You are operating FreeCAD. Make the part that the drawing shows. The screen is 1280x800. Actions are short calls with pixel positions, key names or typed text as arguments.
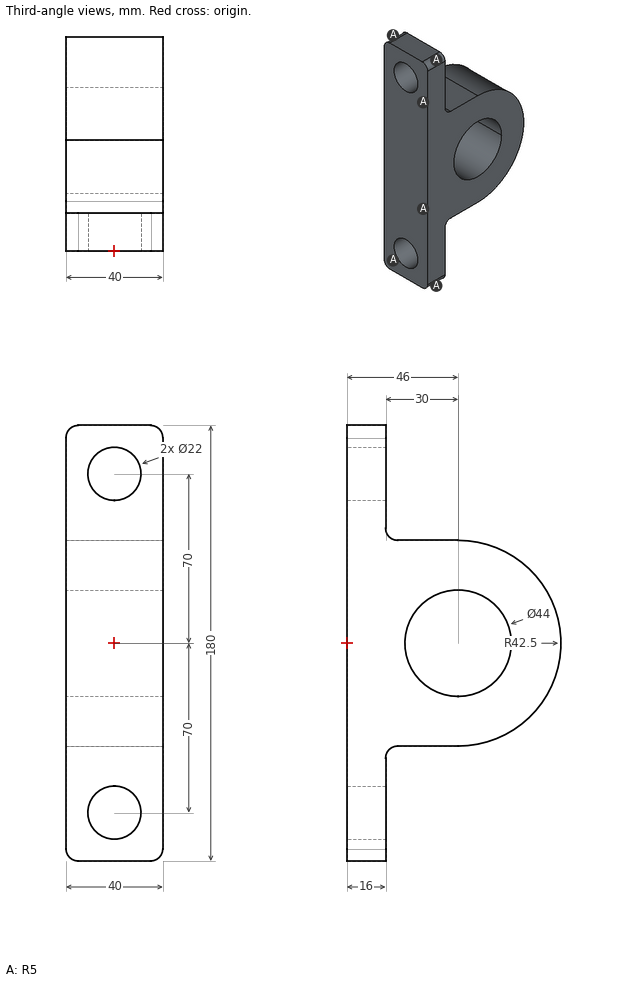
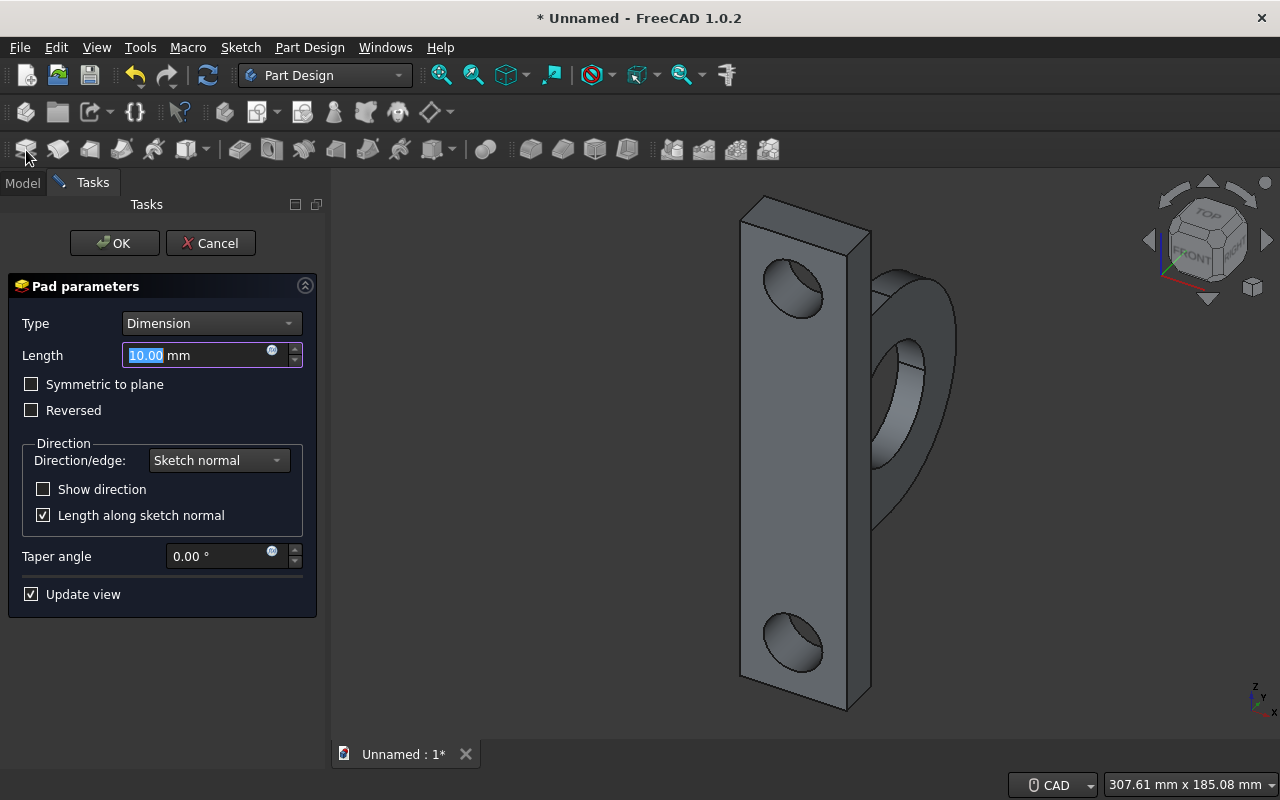
text(40)
key(Tab)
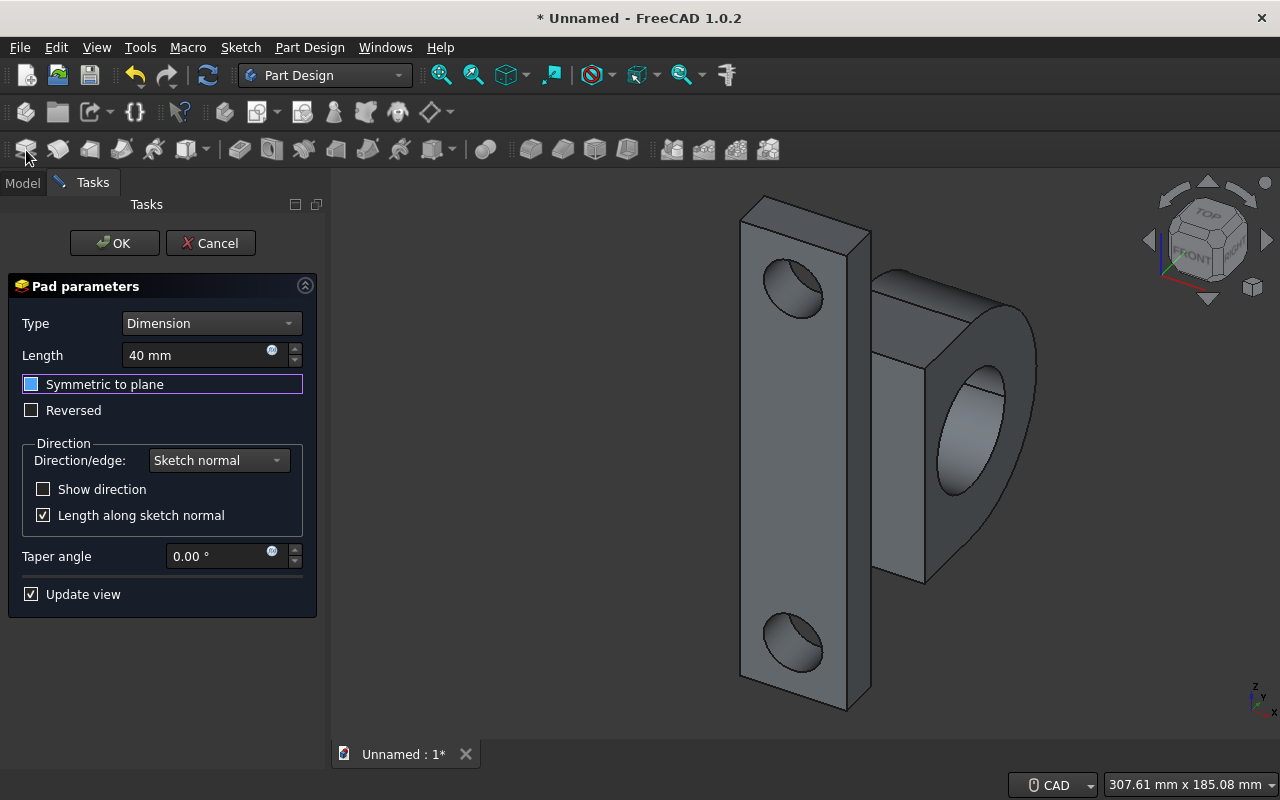
click(30, 384)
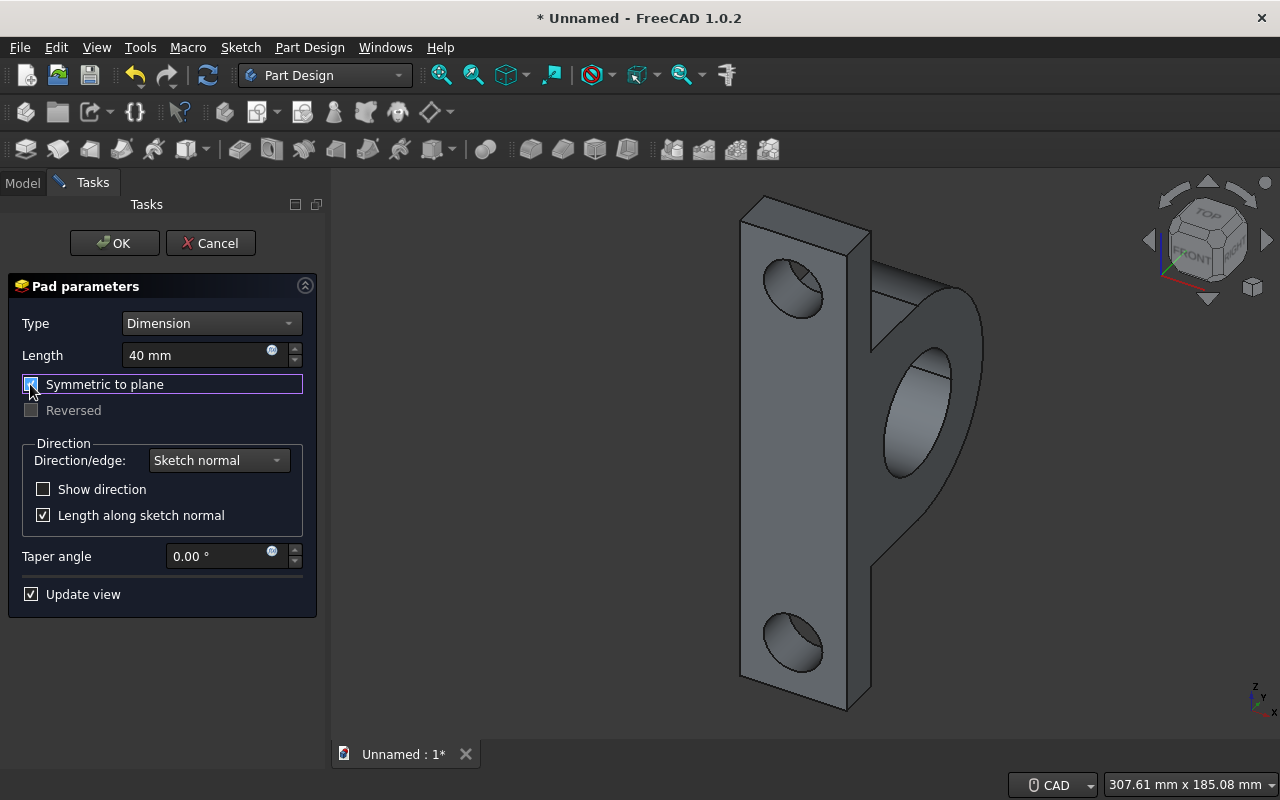
click(115, 243)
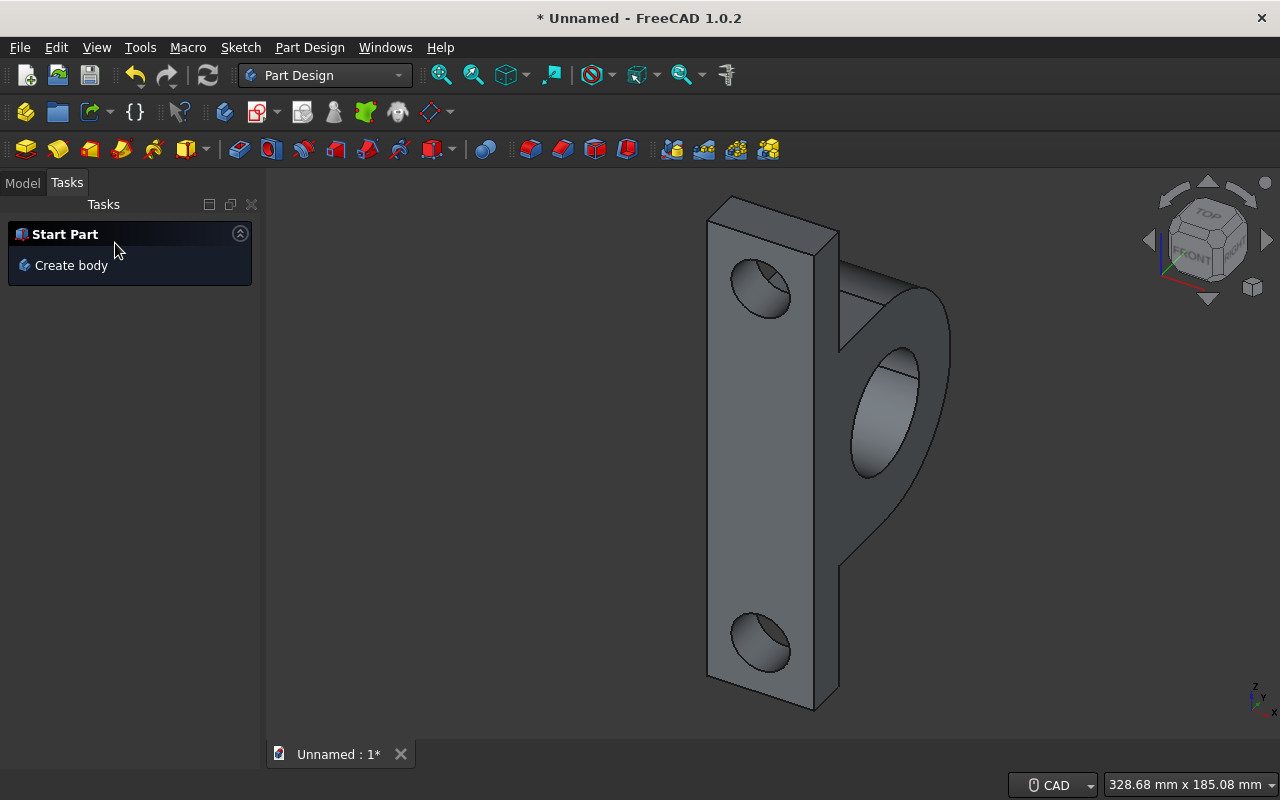
click(442, 76)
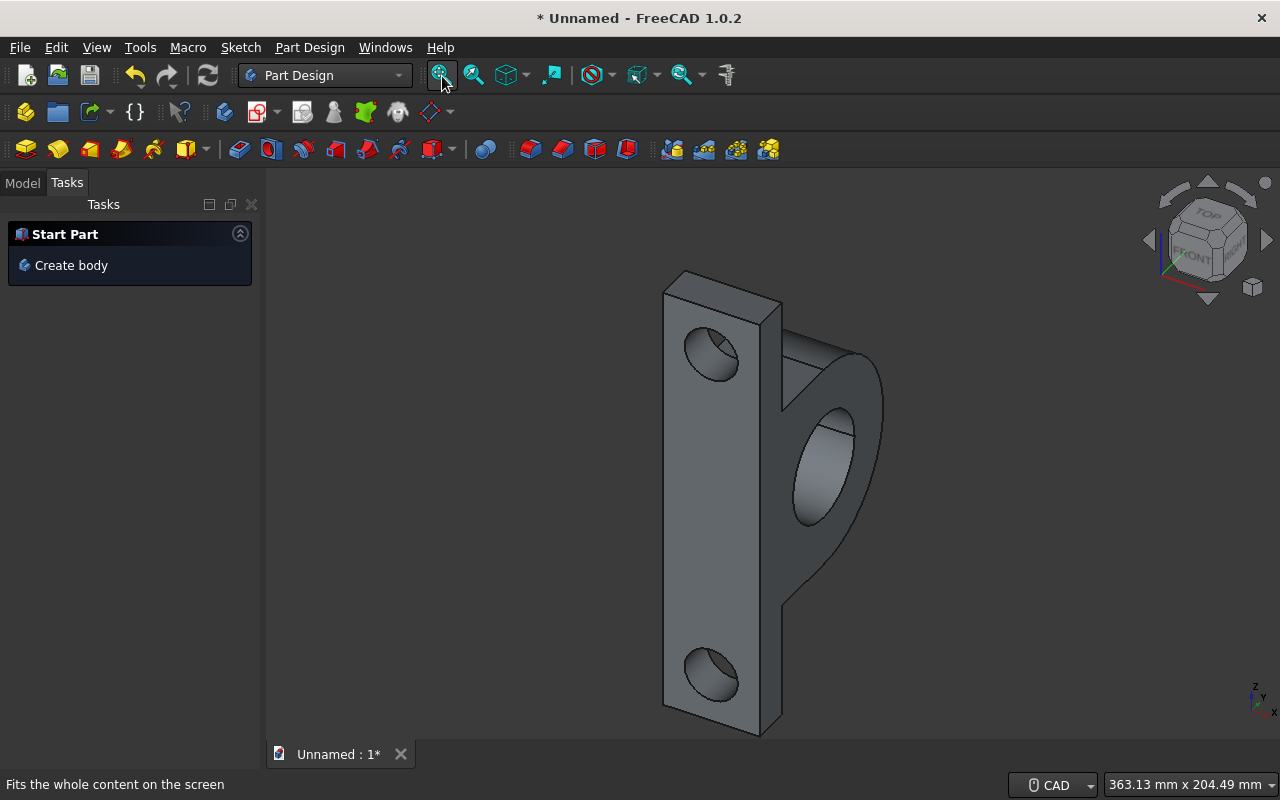
click(771, 313)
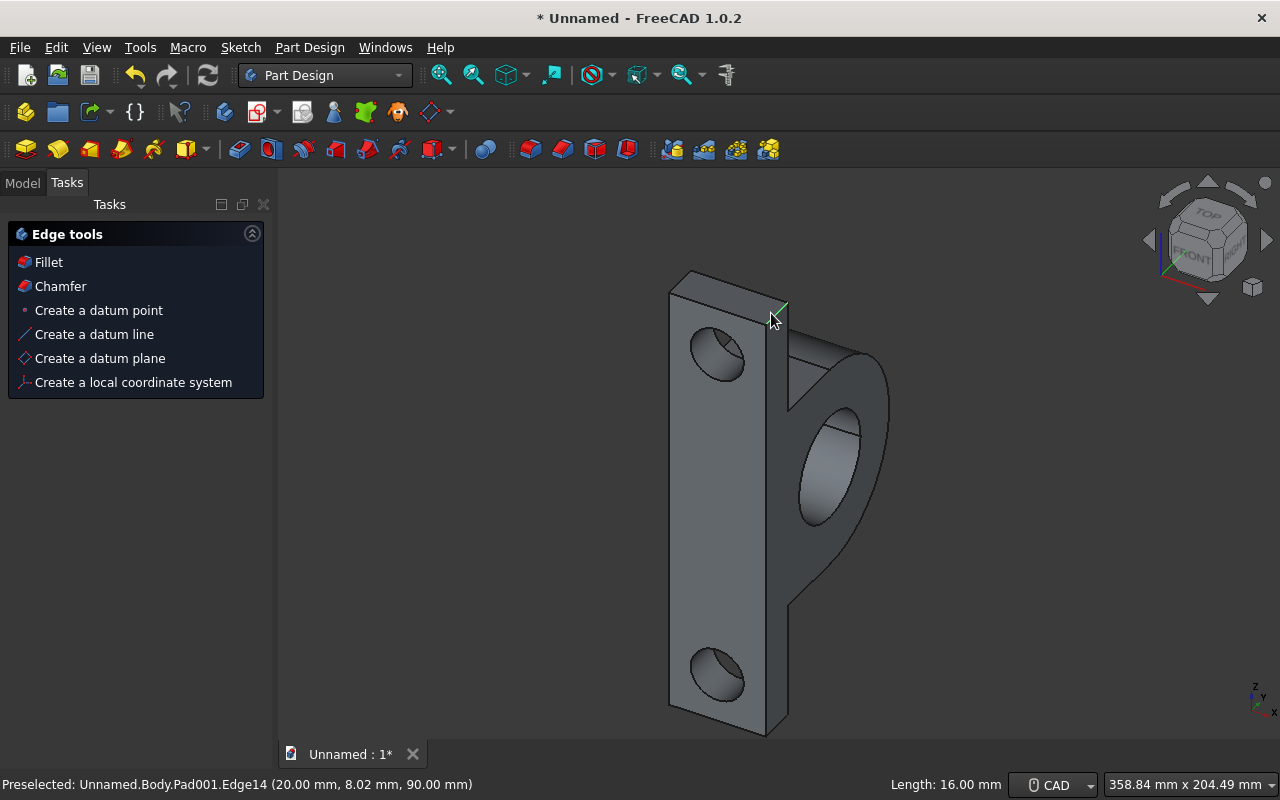
key(0)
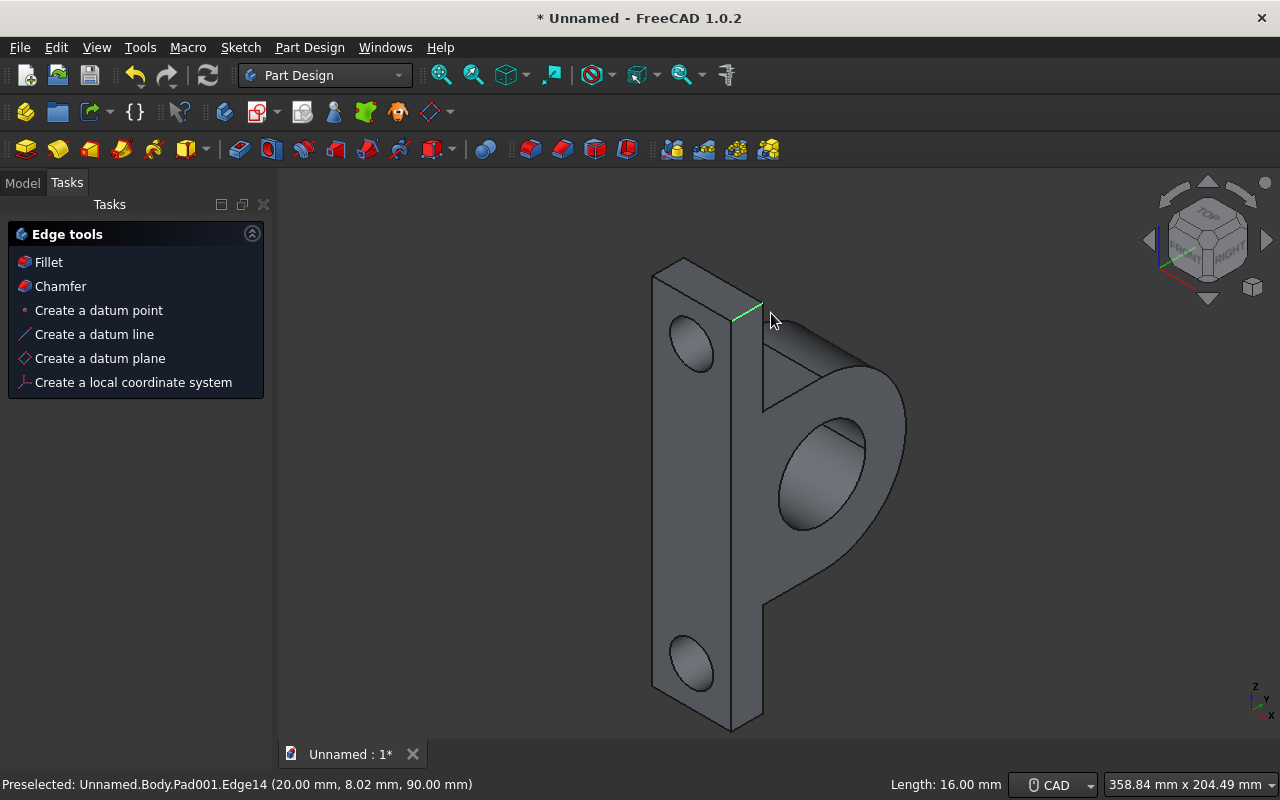
key(2)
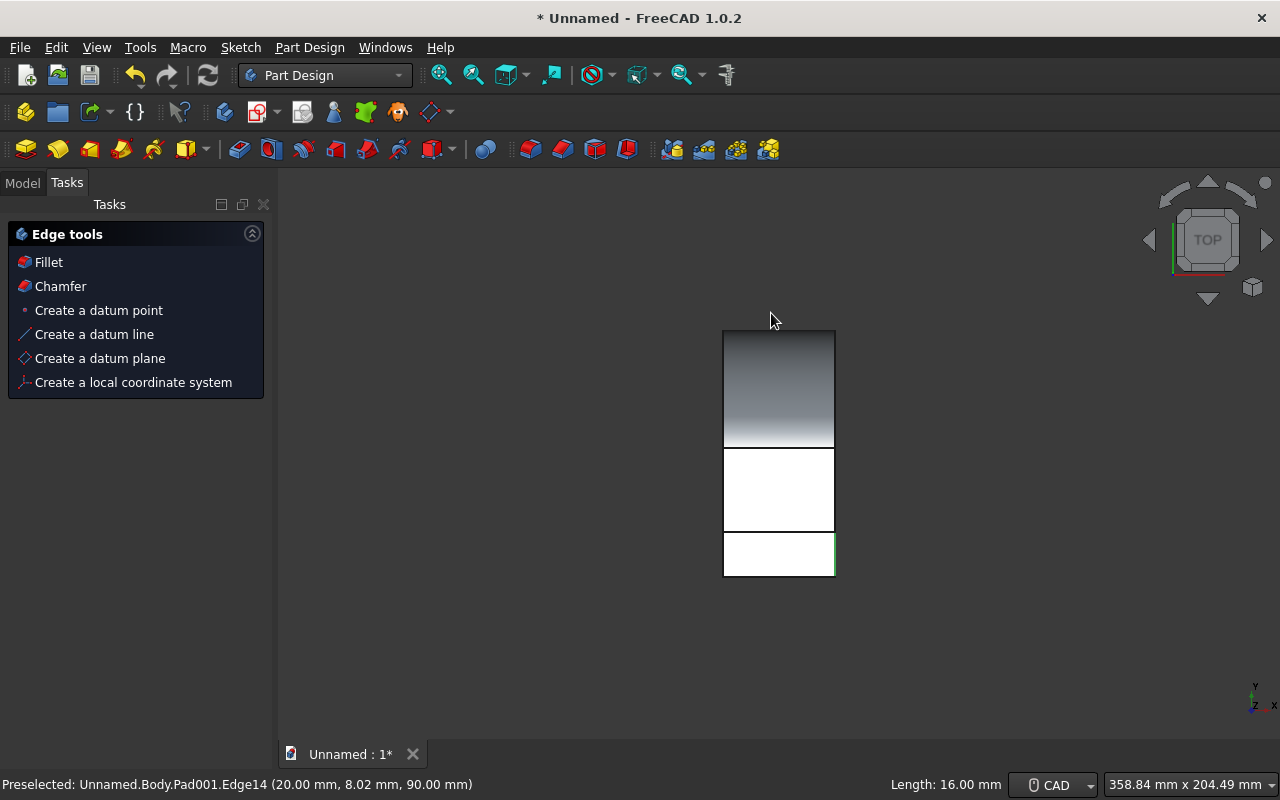
click(442, 76)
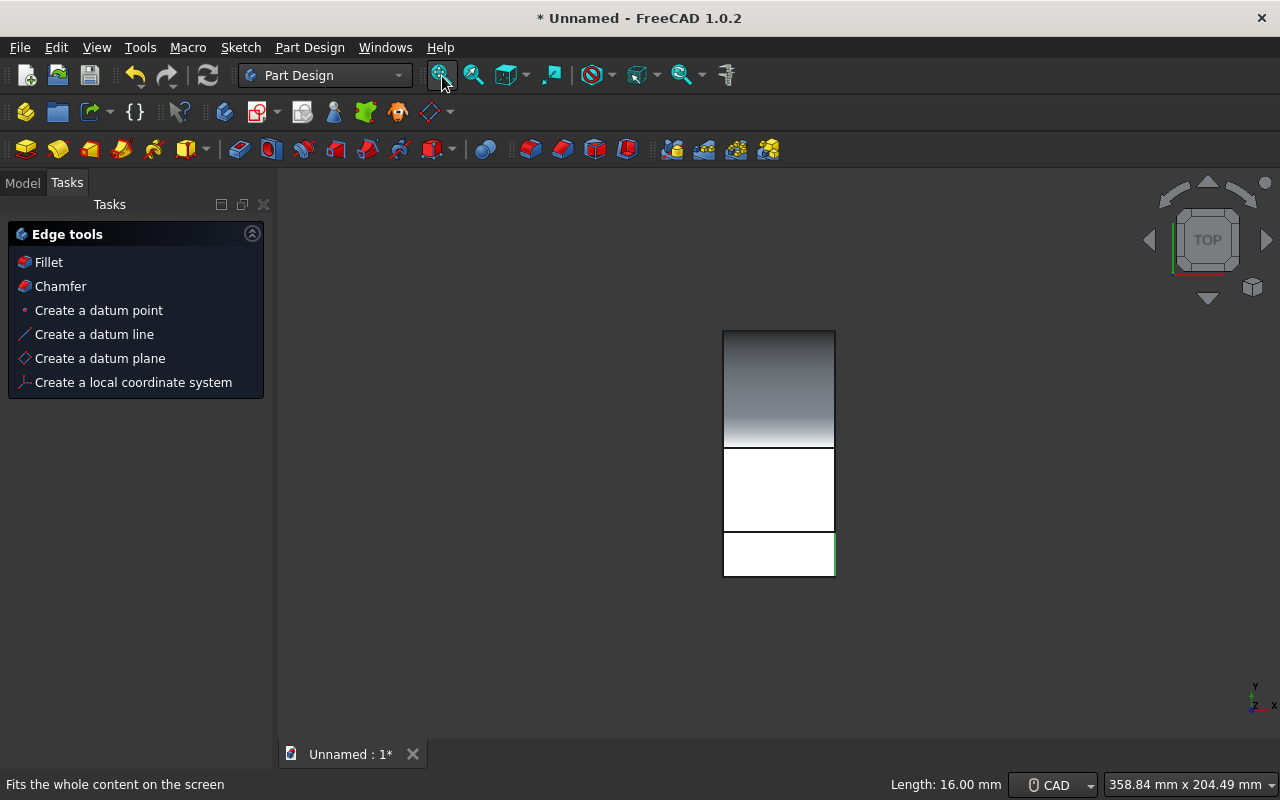
click(723, 554, ctrl)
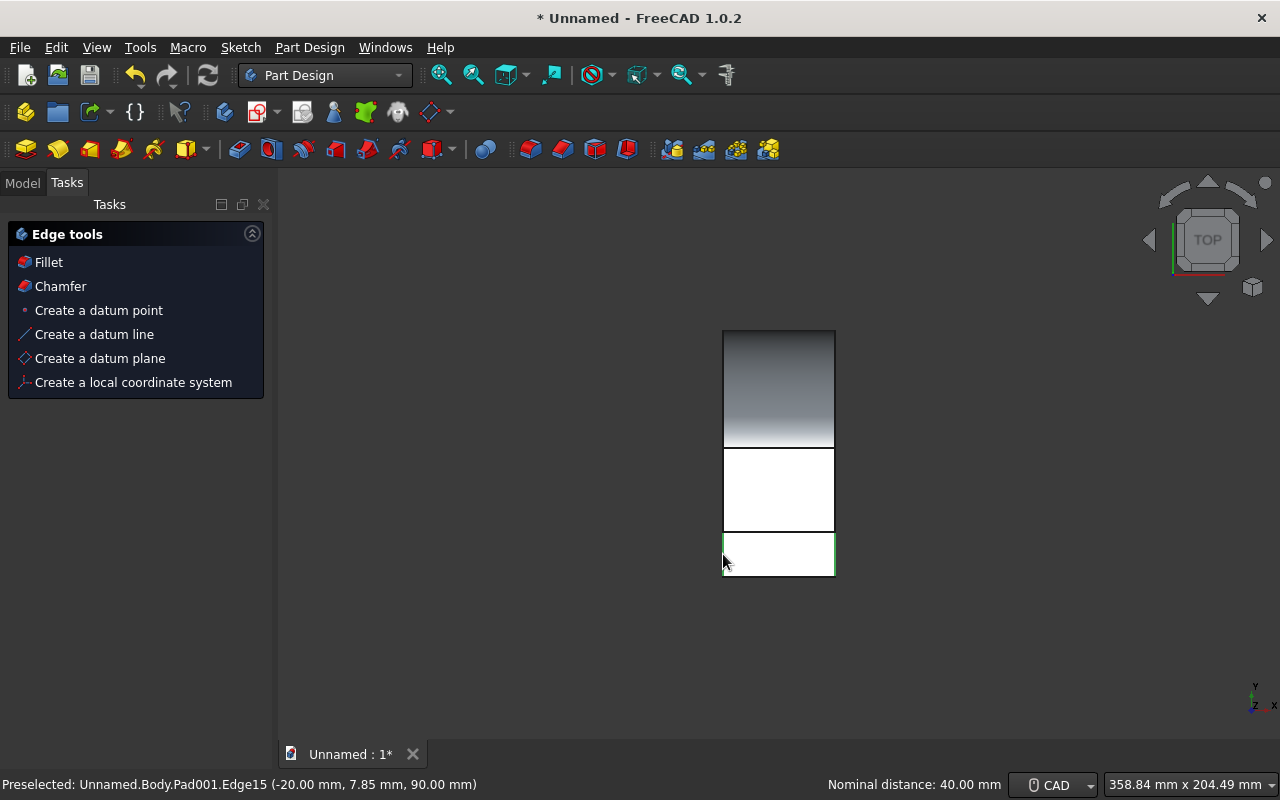
key(1)